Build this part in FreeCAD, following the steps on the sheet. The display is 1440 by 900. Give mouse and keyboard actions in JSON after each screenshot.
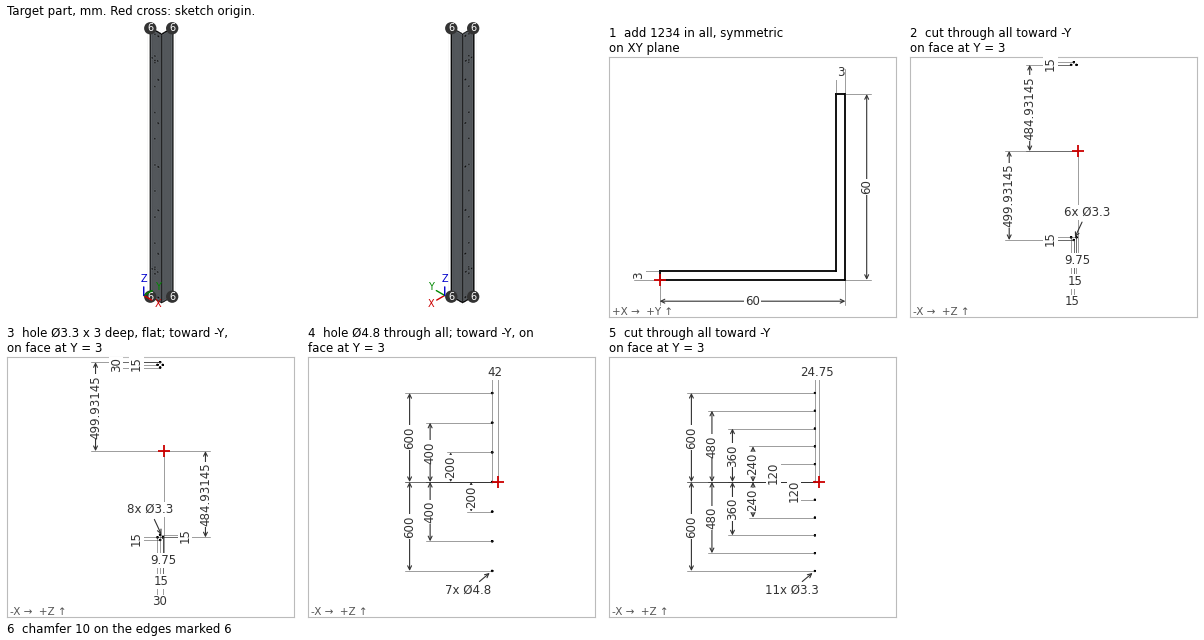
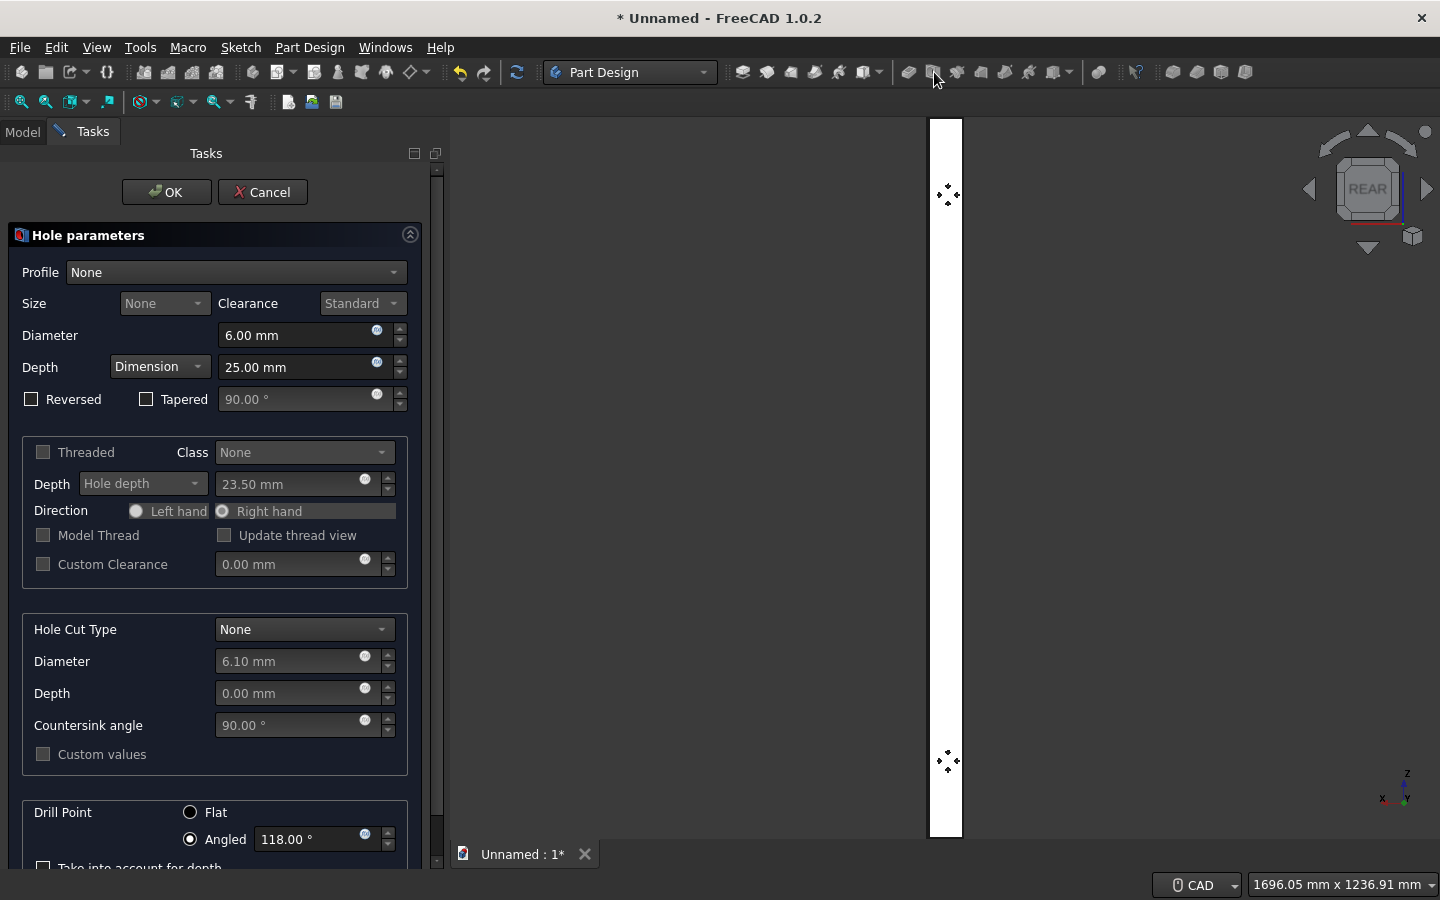
{"action": "triple_click", "coordinate": [305, 335]}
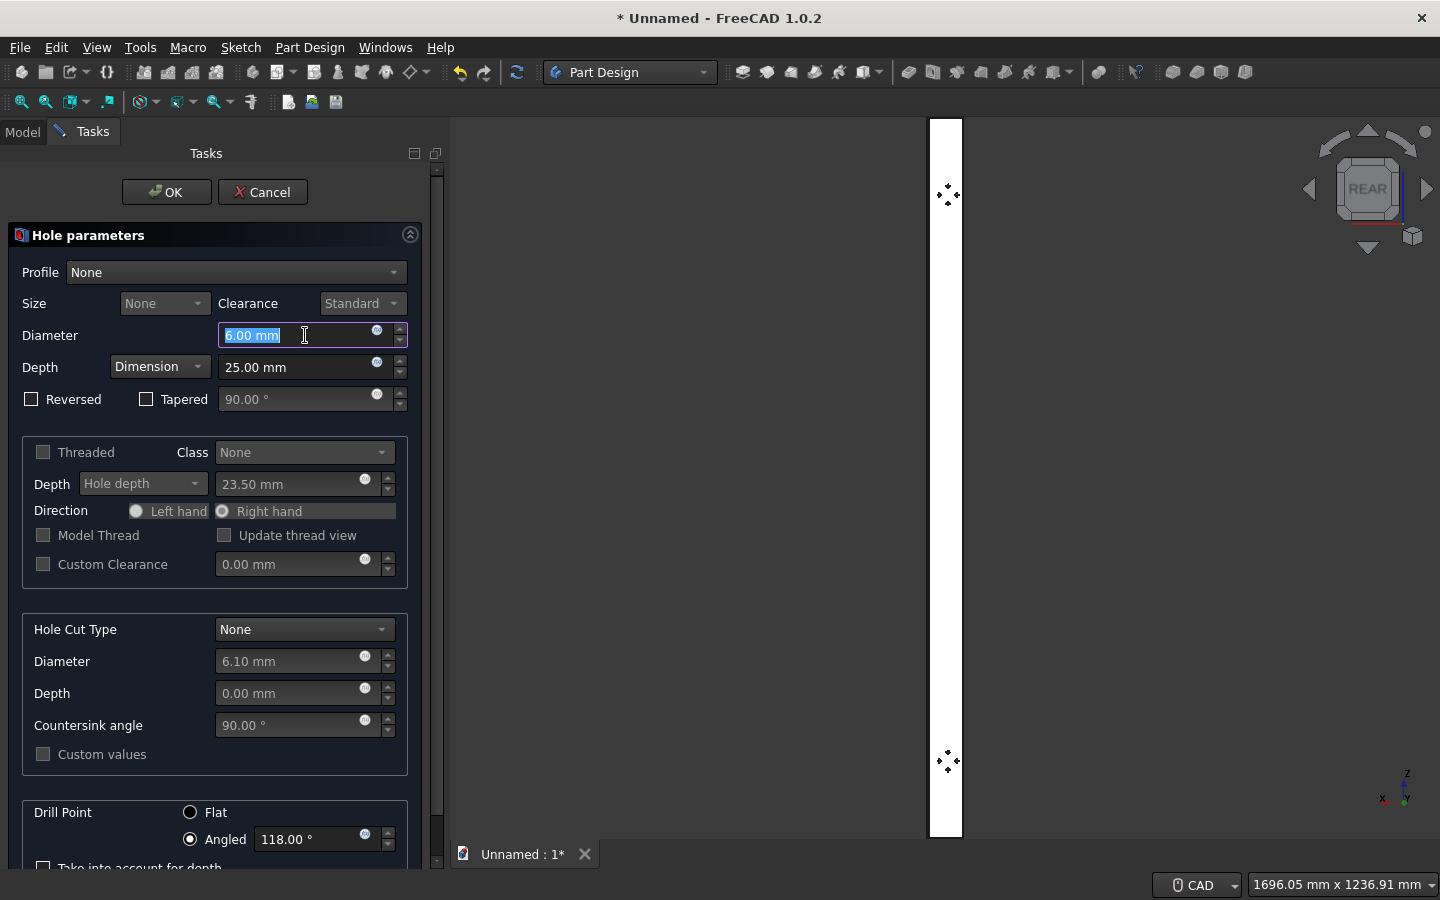
{"action": "type", "text": "3.3"}
{"action": "key", "text": "Tab"}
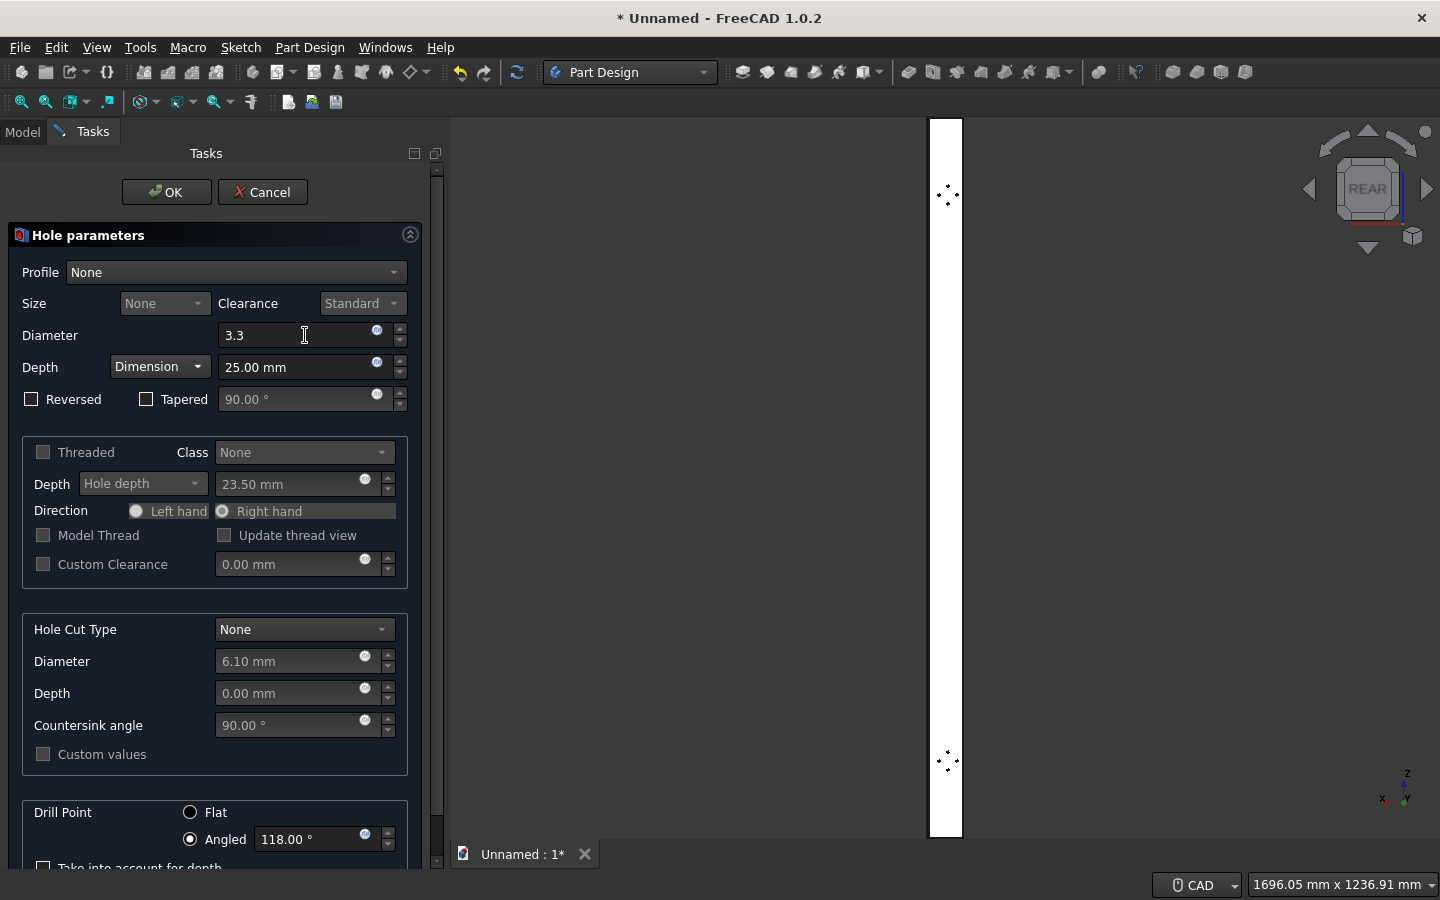
{"action": "triple_click", "coordinate": [305, 367]}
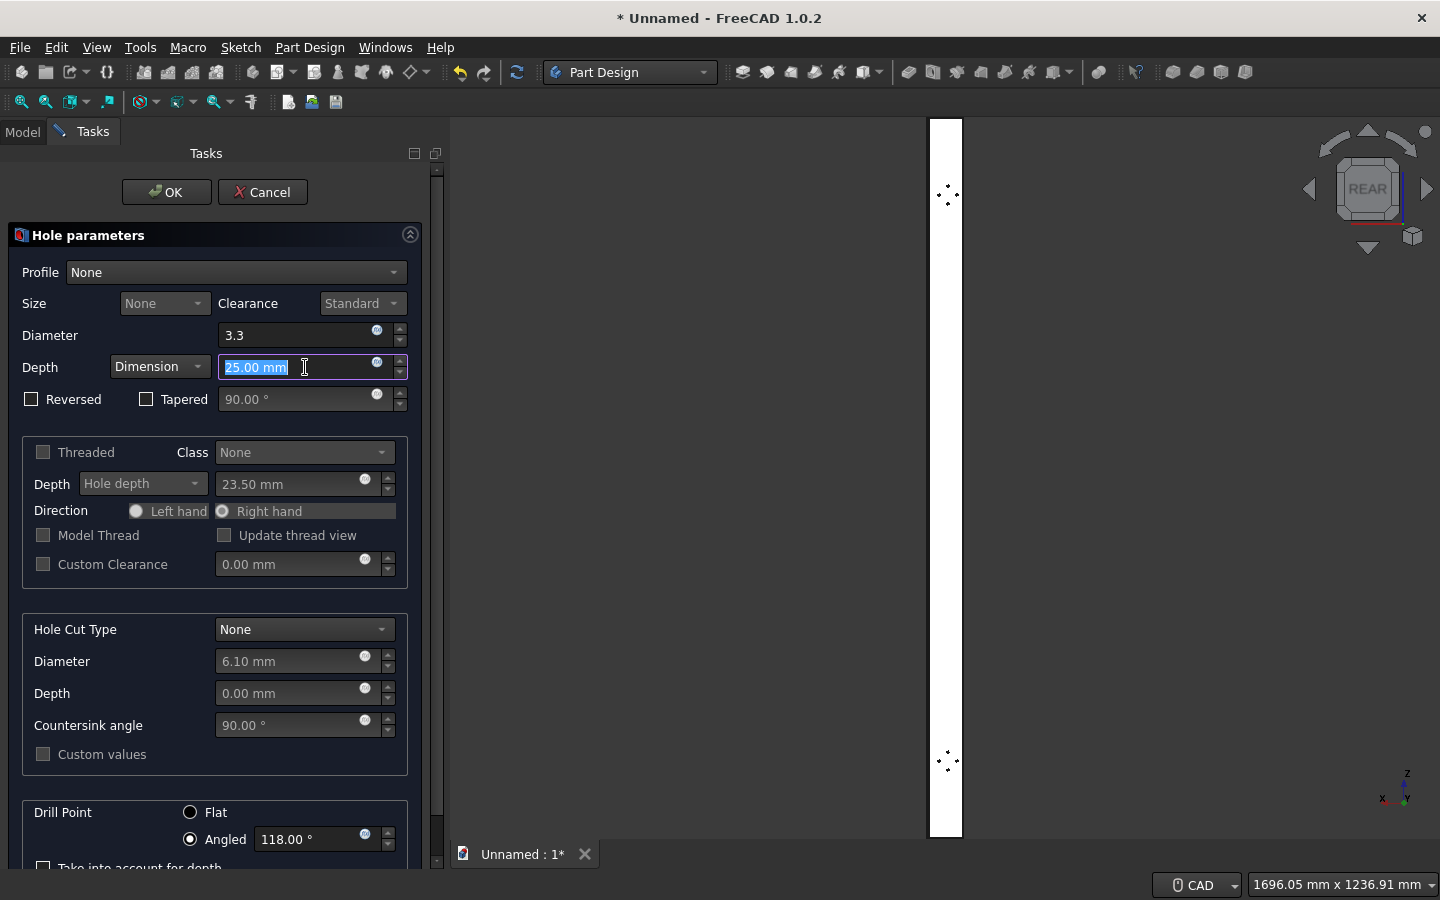
{"action": "type", "text": "3"}
{"action": "key", "text": "Tab"}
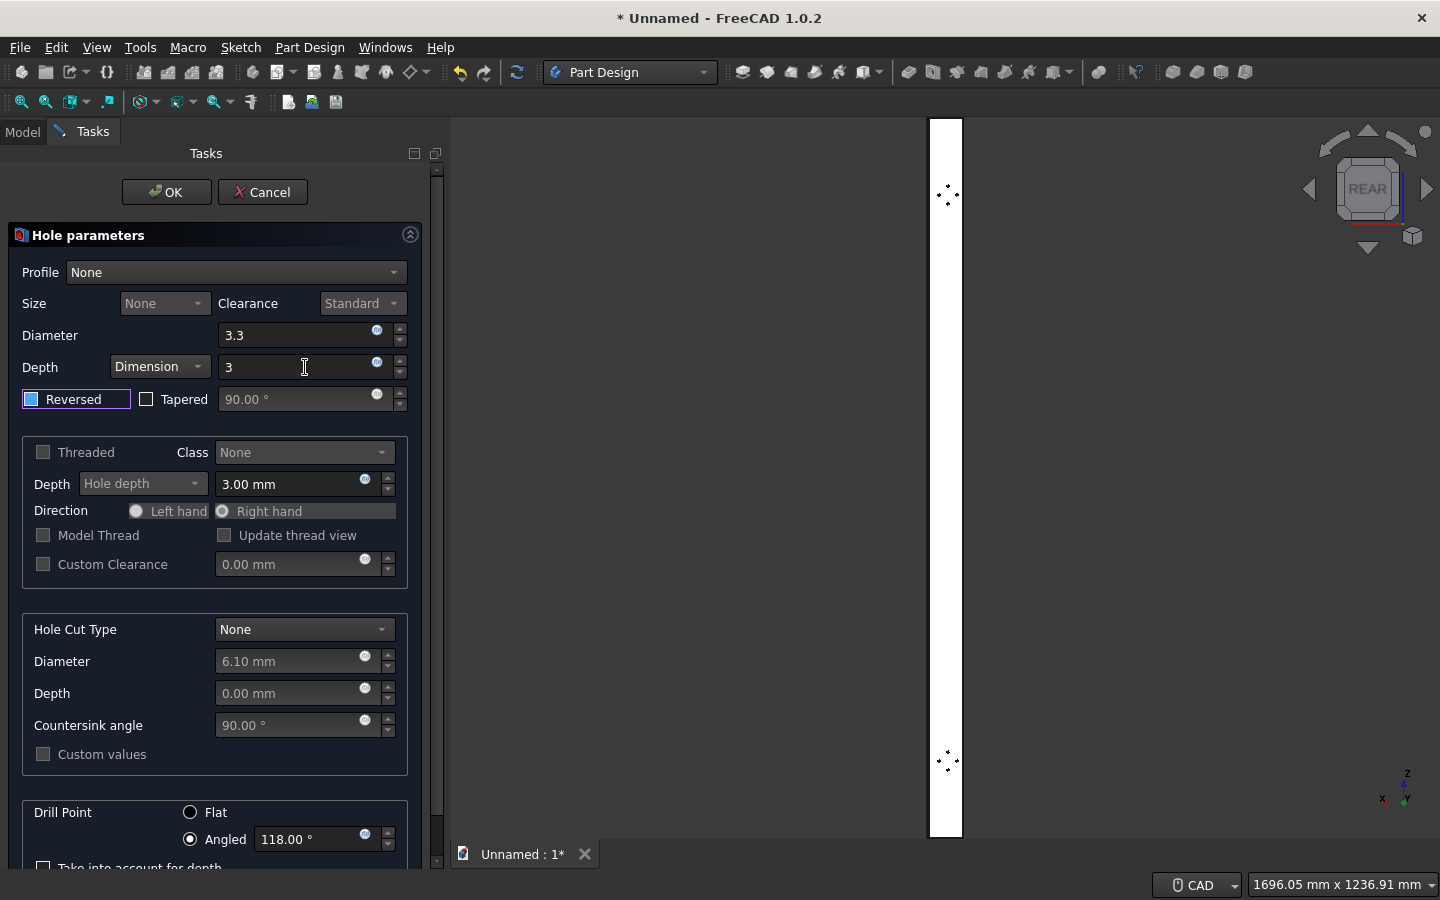
{"action": "left_click", "coordinate": [191, 812]}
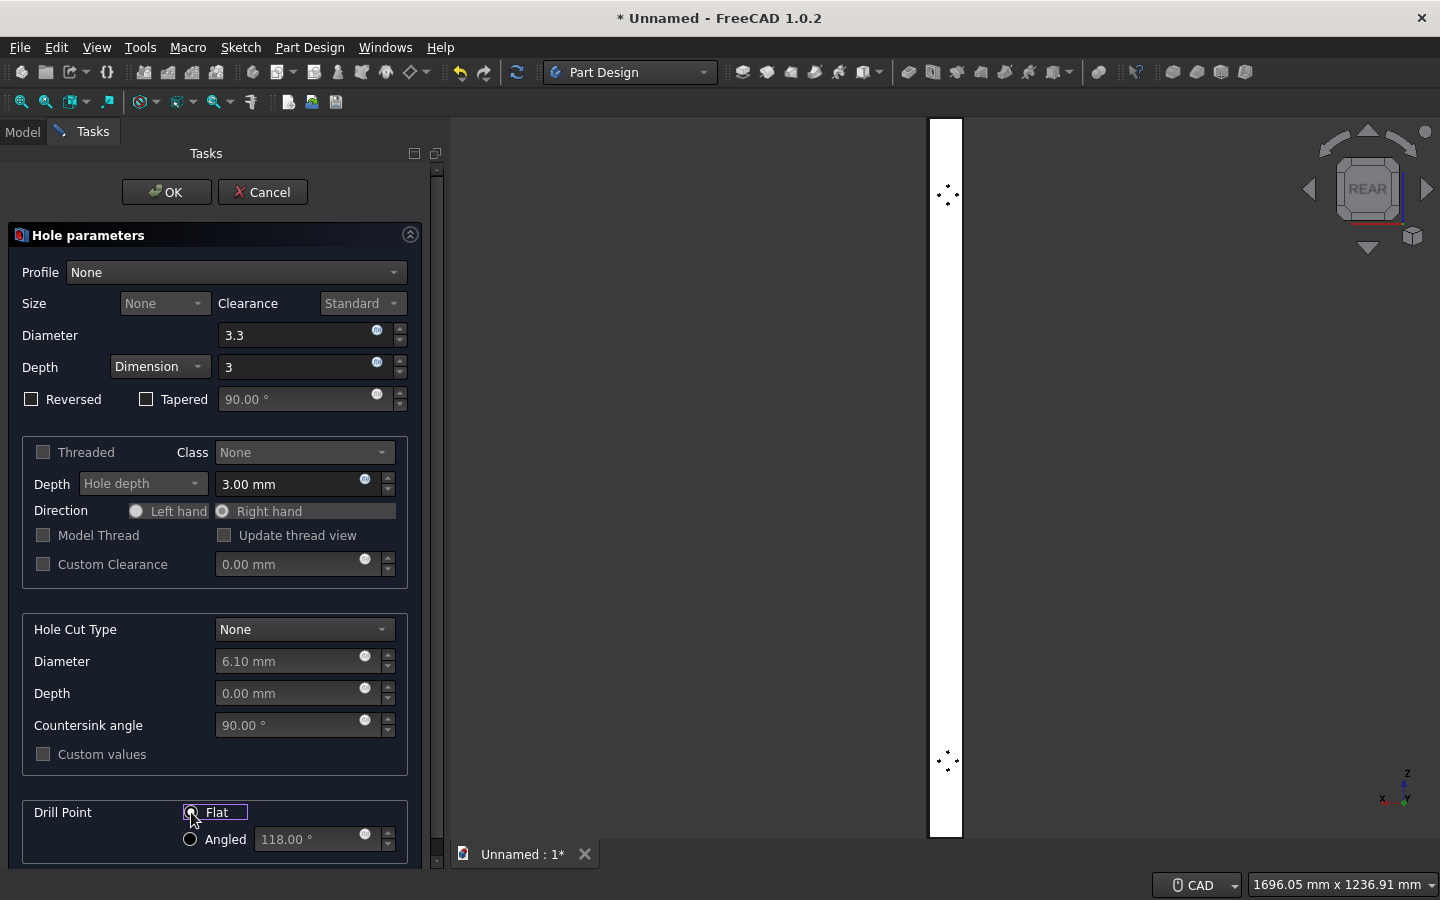
{"action": "left_click", "coordinate": [167, 192]}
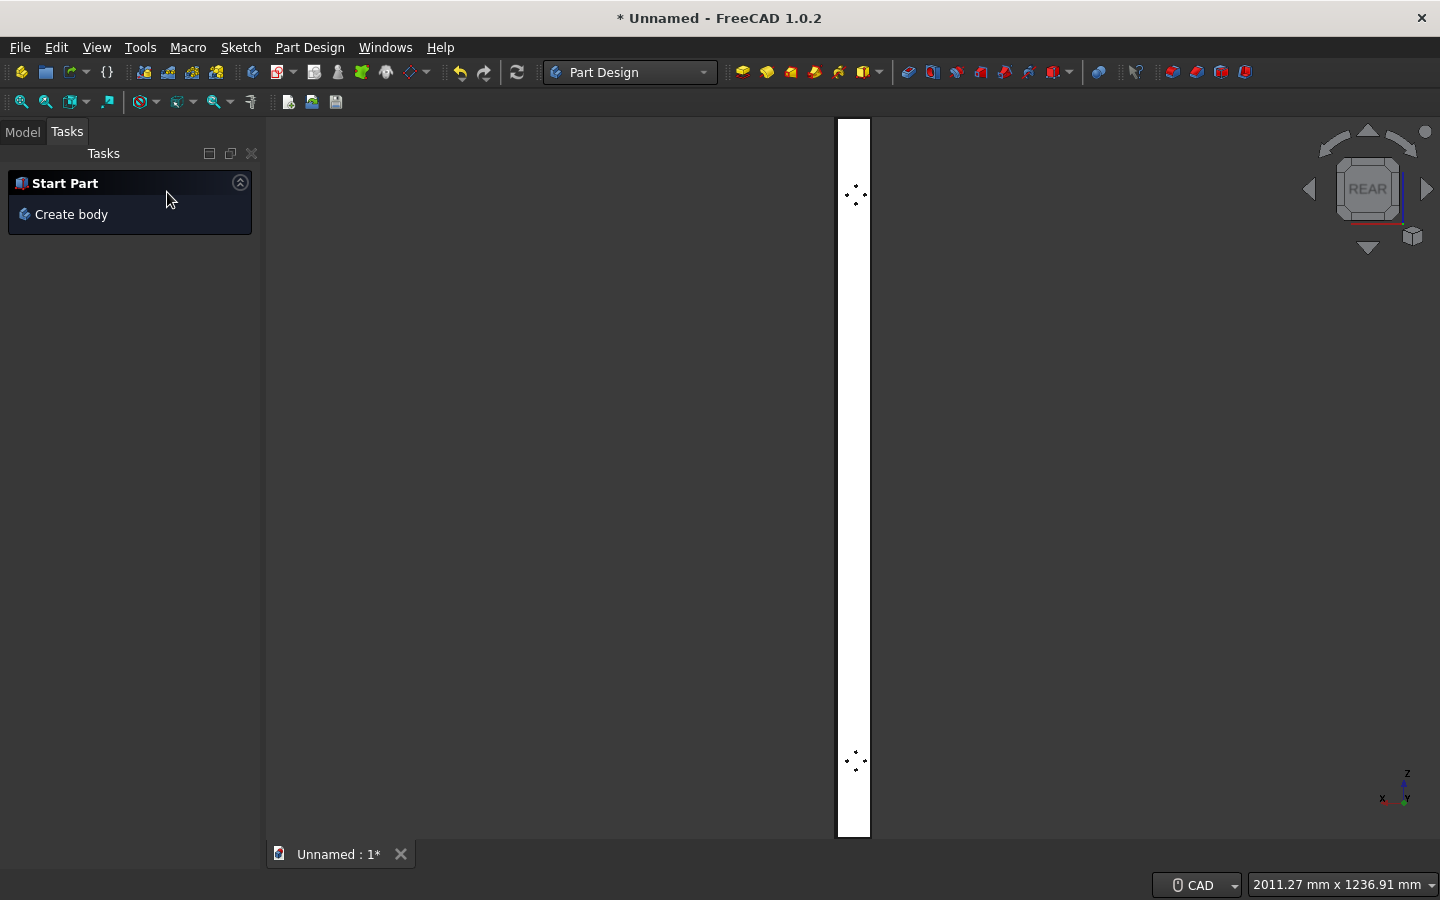
{"action": "left_click", "coordinate": [854, 271]}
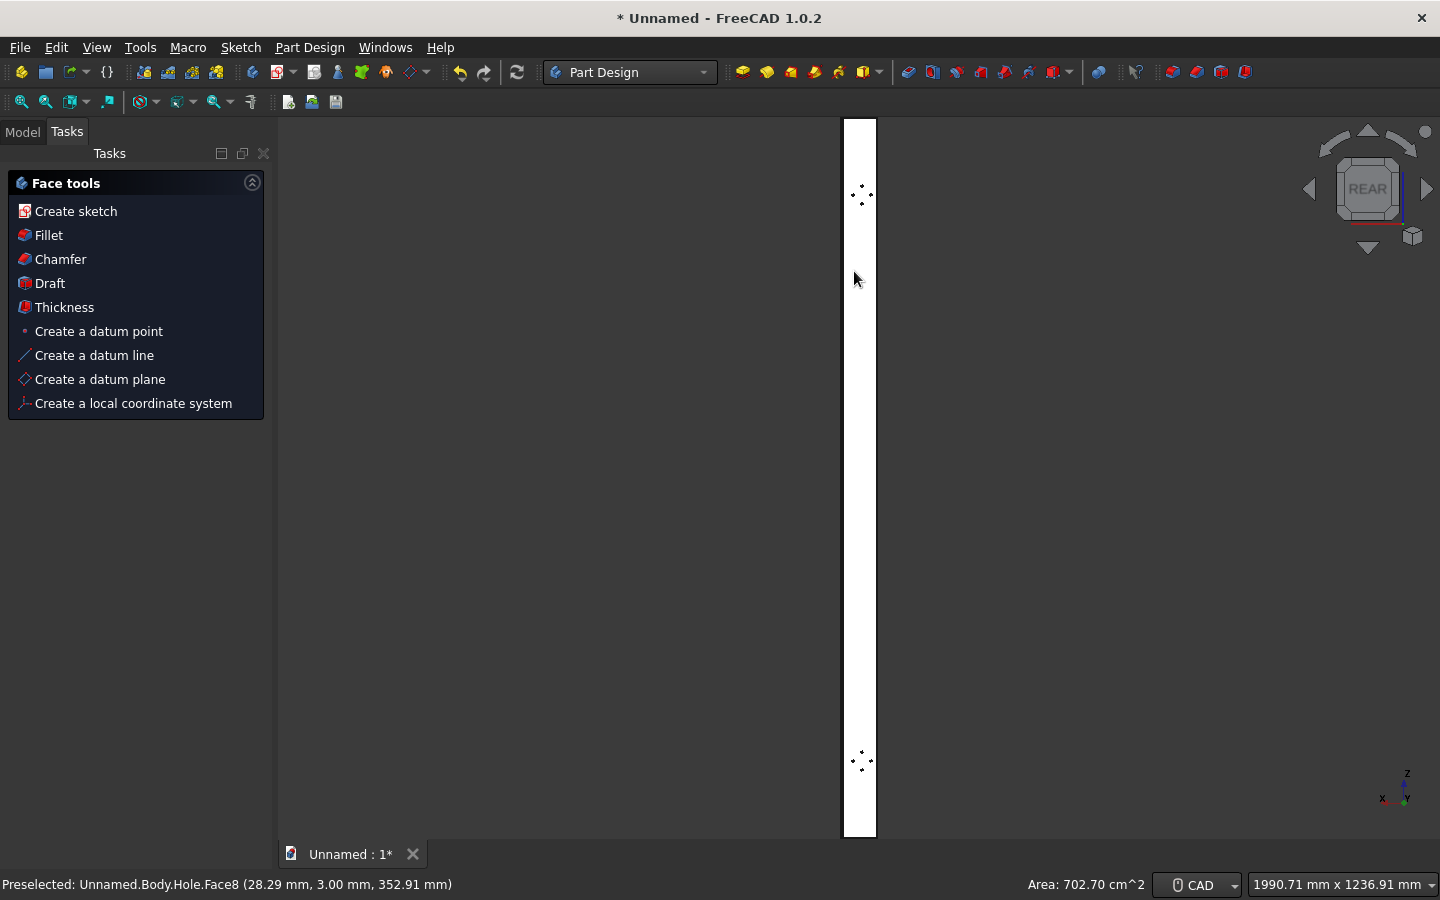
{"action": "left_click", "coordinate": [278, 72]}